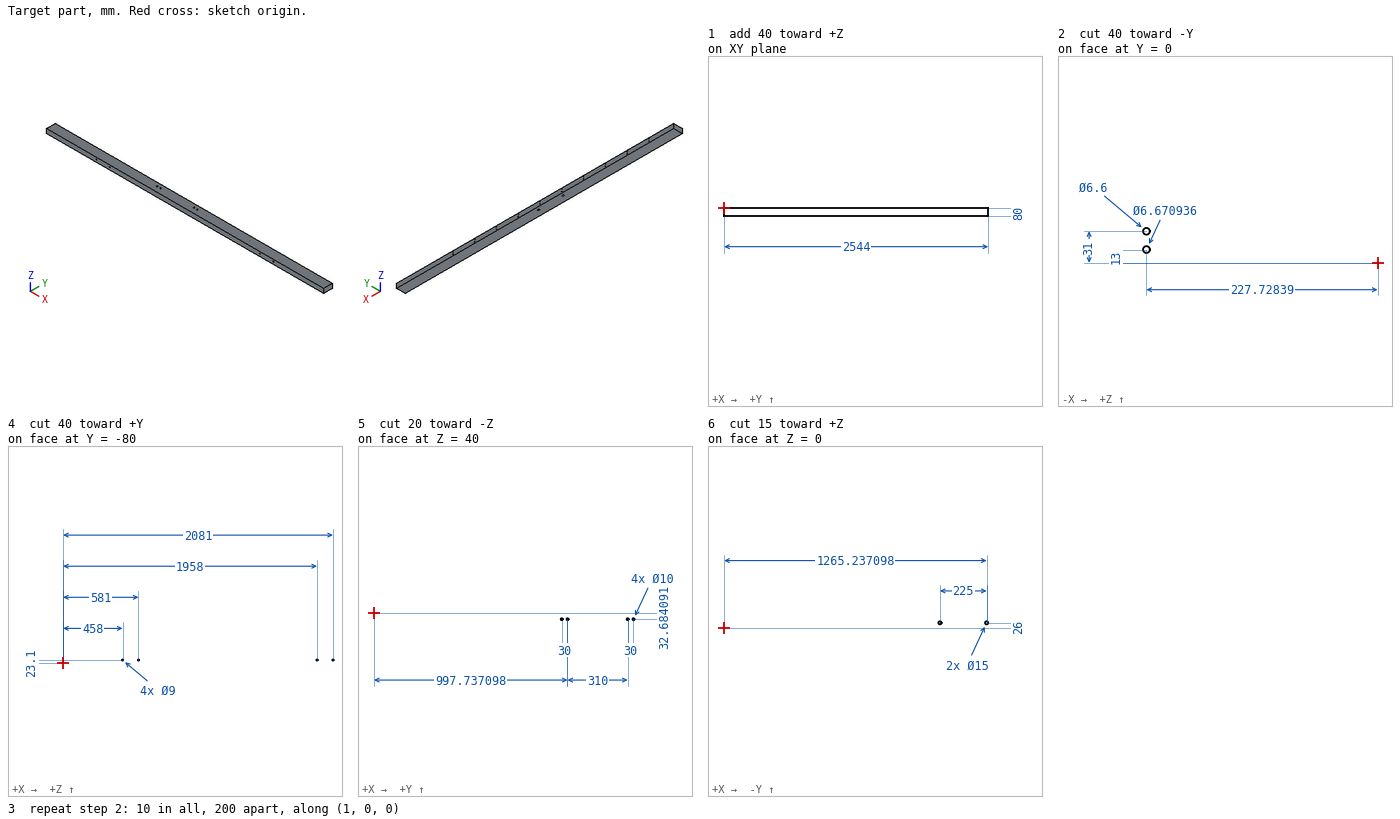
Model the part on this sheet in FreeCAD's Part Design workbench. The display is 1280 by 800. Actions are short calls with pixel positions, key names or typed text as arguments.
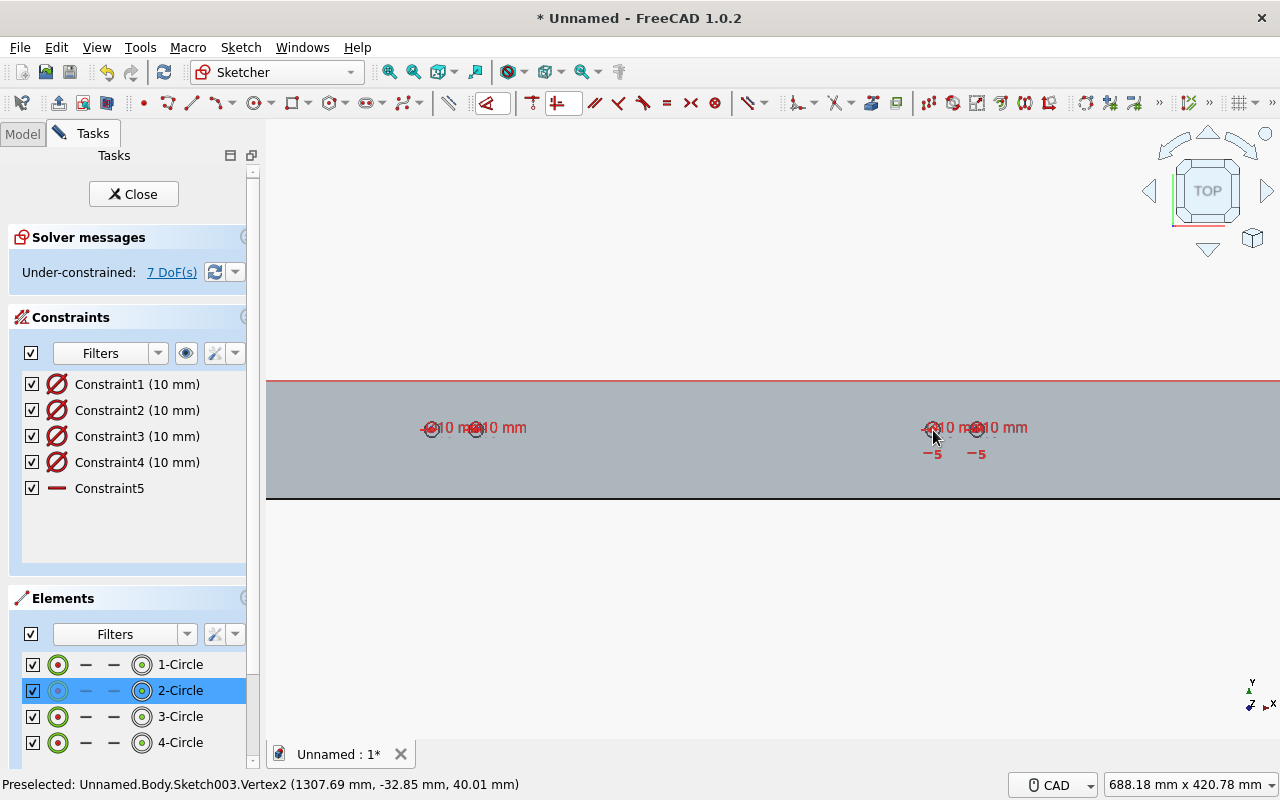
click(476, 430)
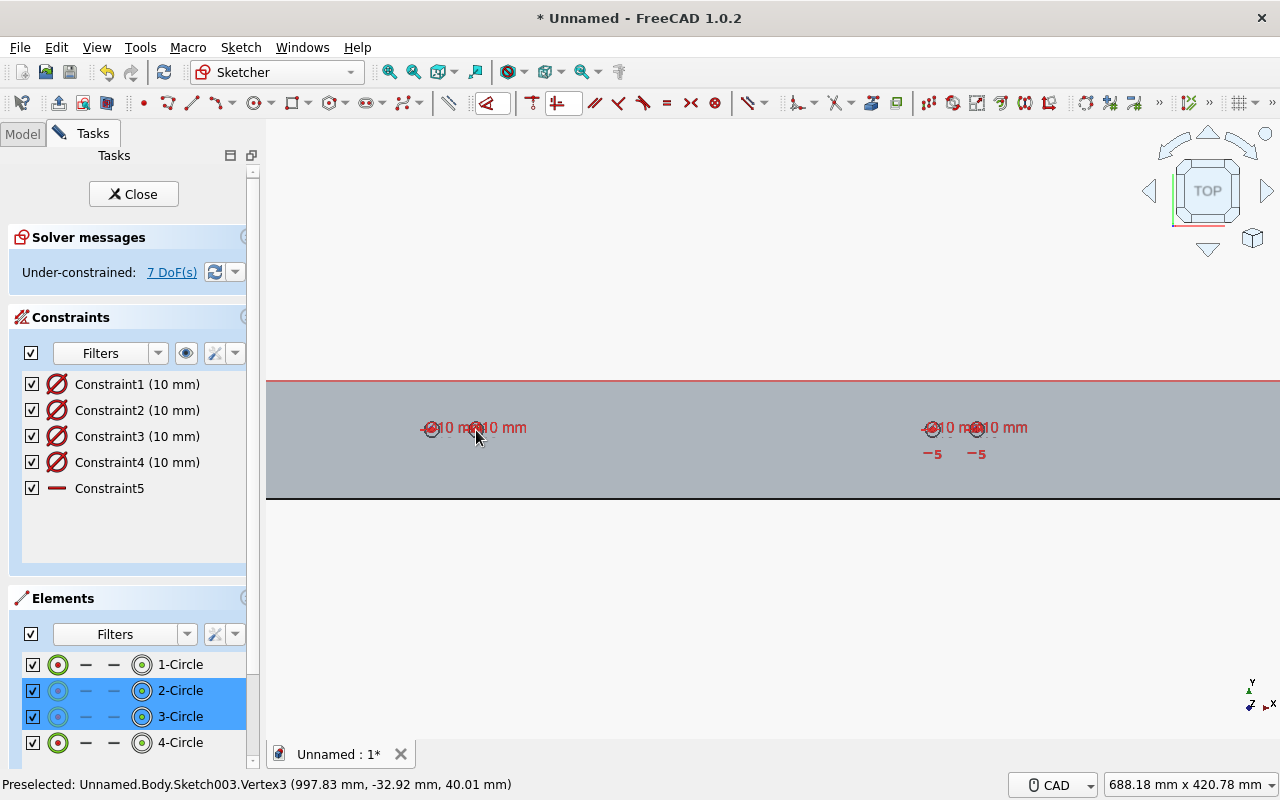
click(576, 104)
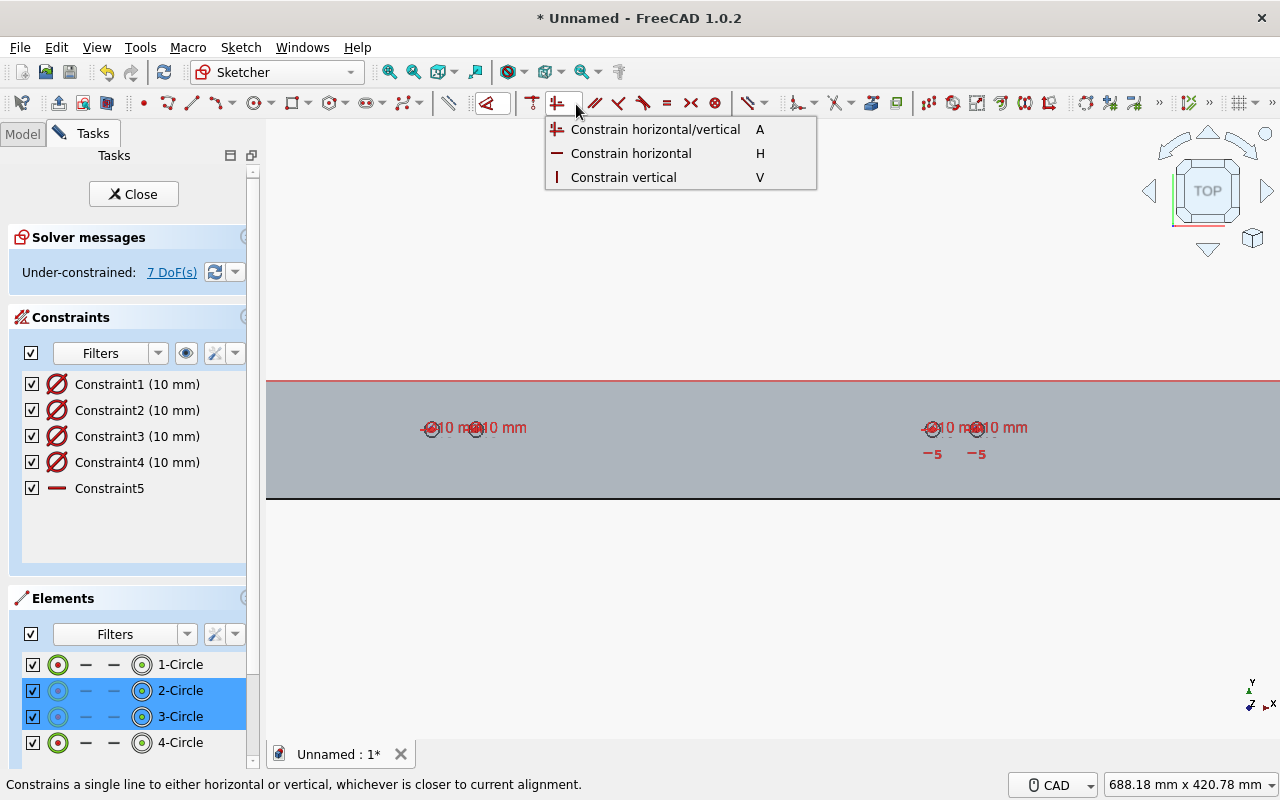
click(681, 153)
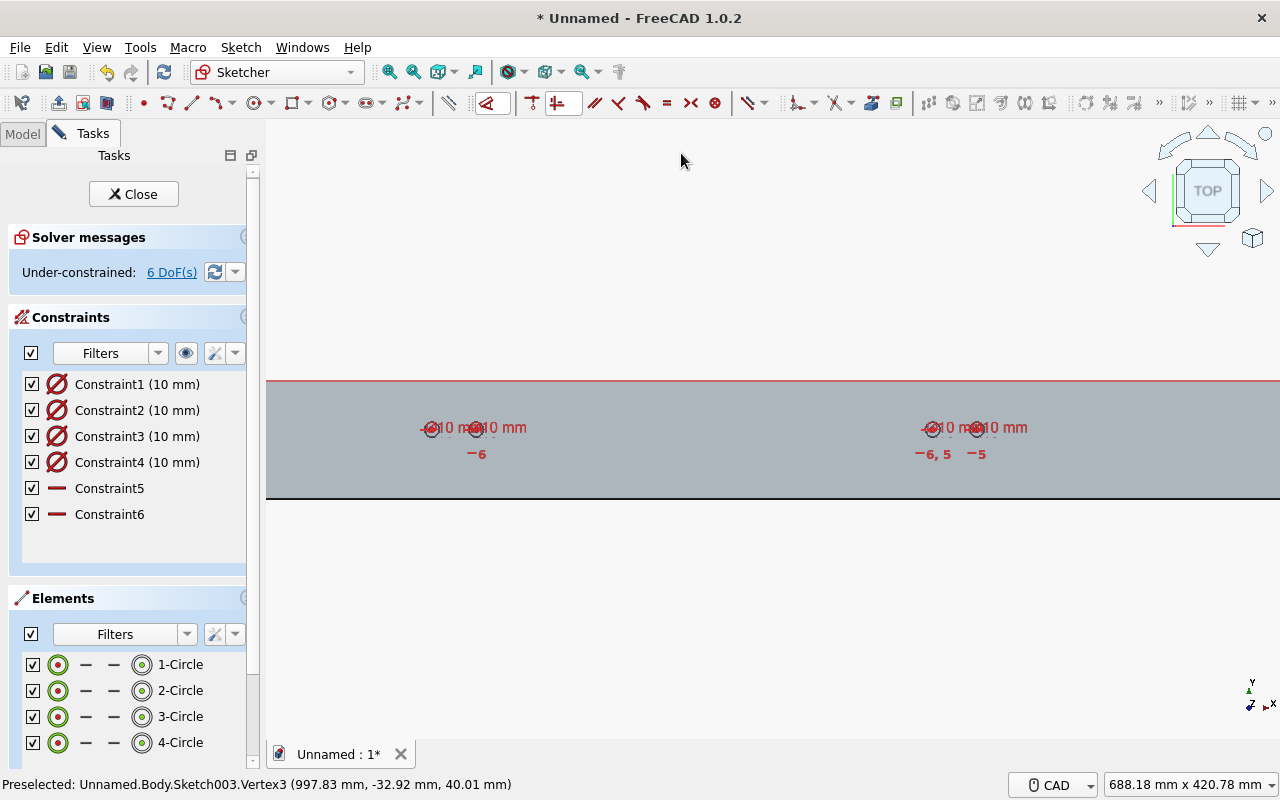
click(476, 430)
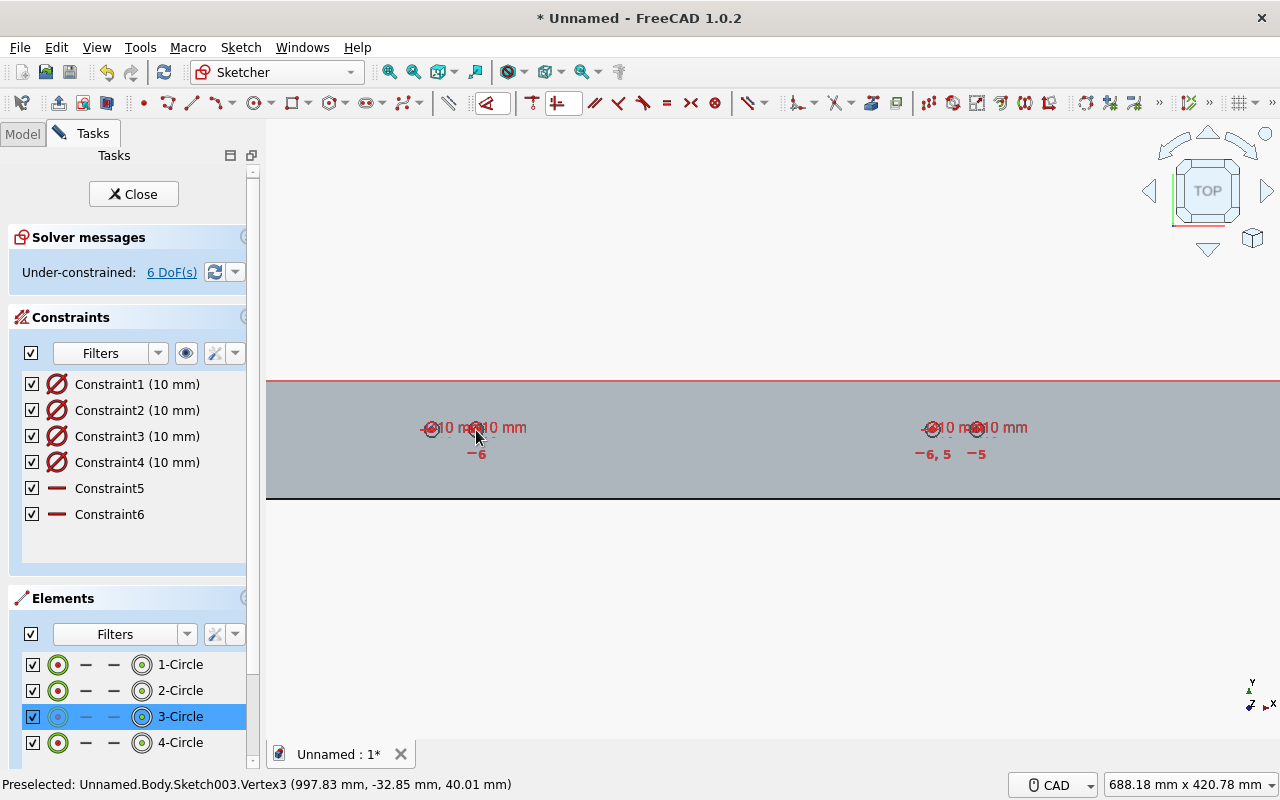
click(432, 430)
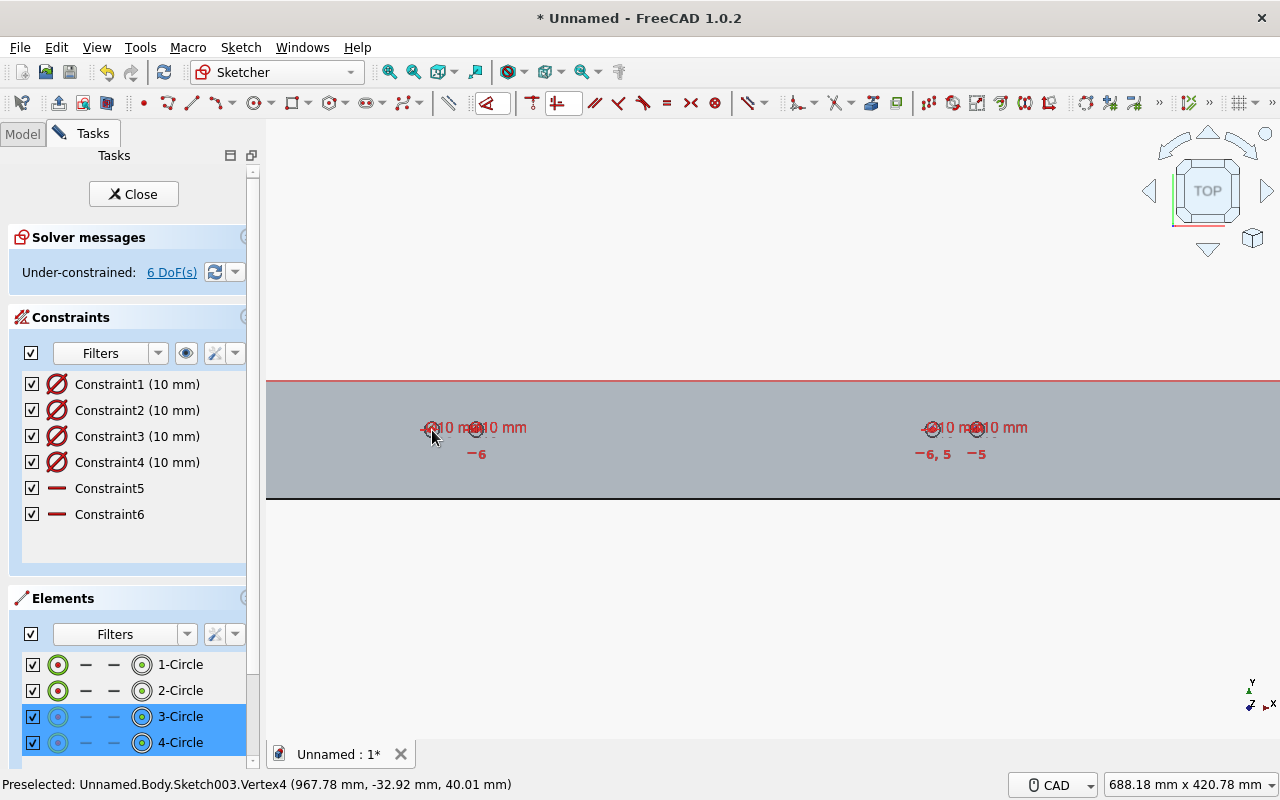
click(576, 104)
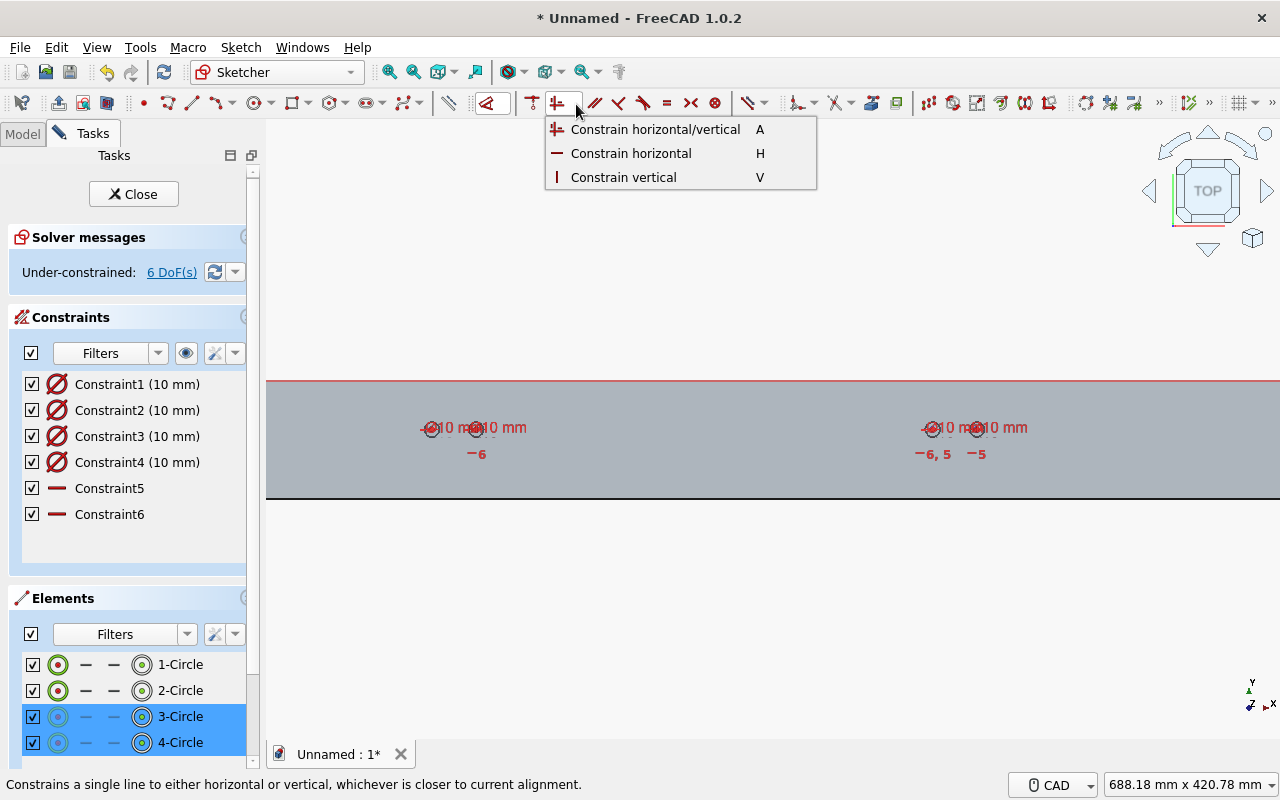
click(681, 153)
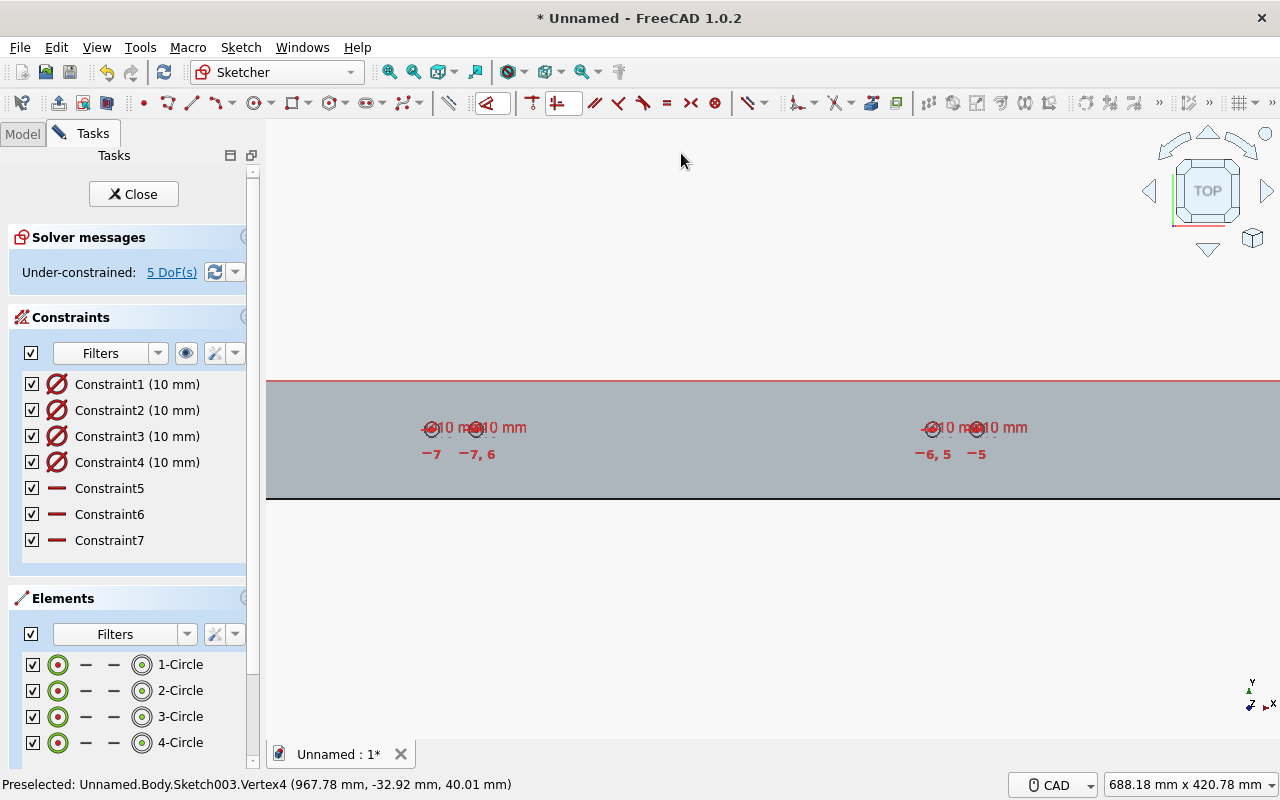
key(d)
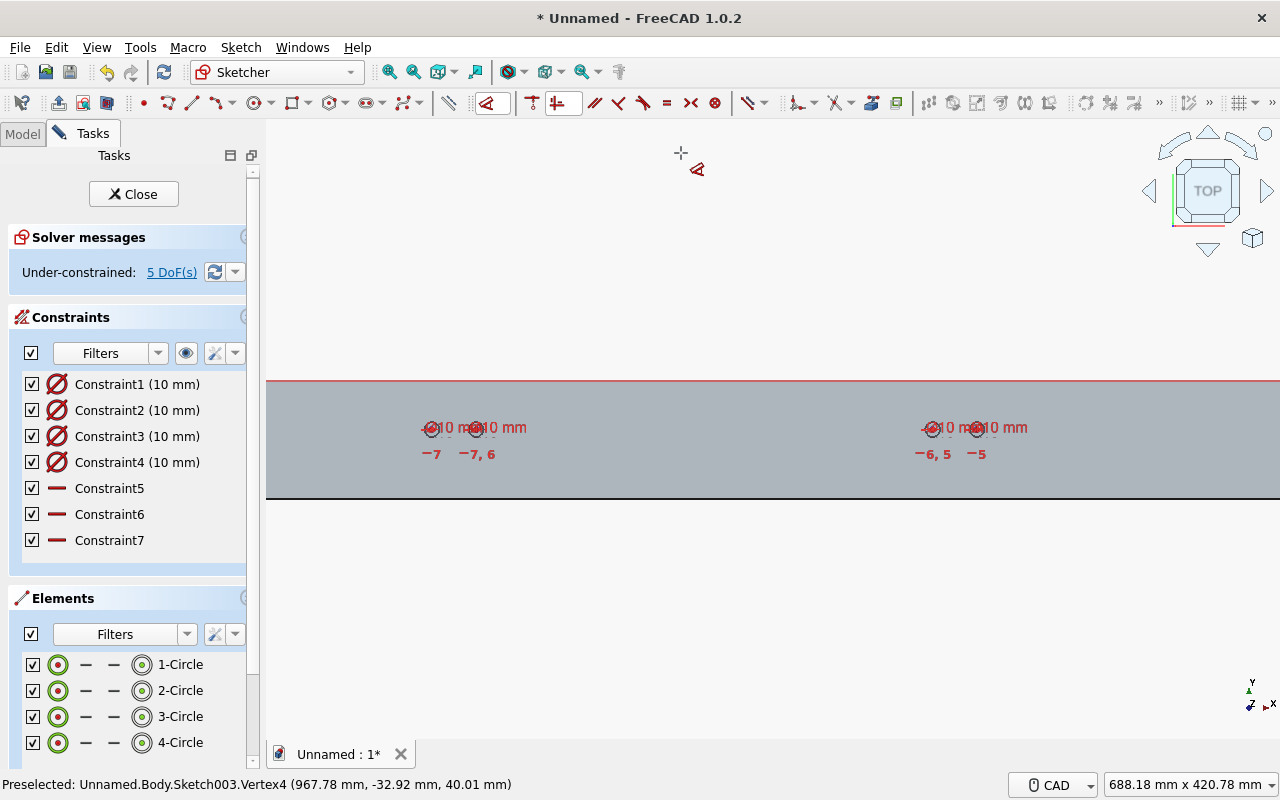
click(977, 430)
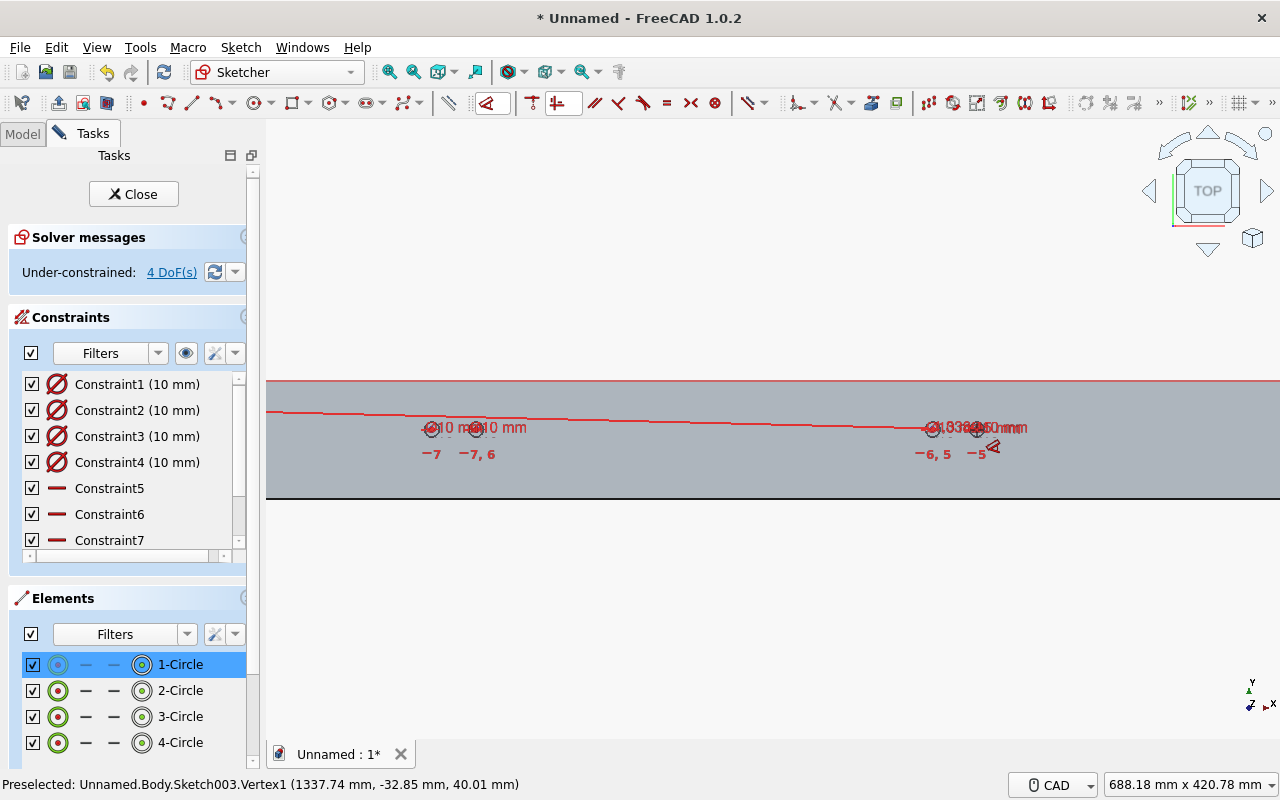
click(933, 430)
click(955, 464)